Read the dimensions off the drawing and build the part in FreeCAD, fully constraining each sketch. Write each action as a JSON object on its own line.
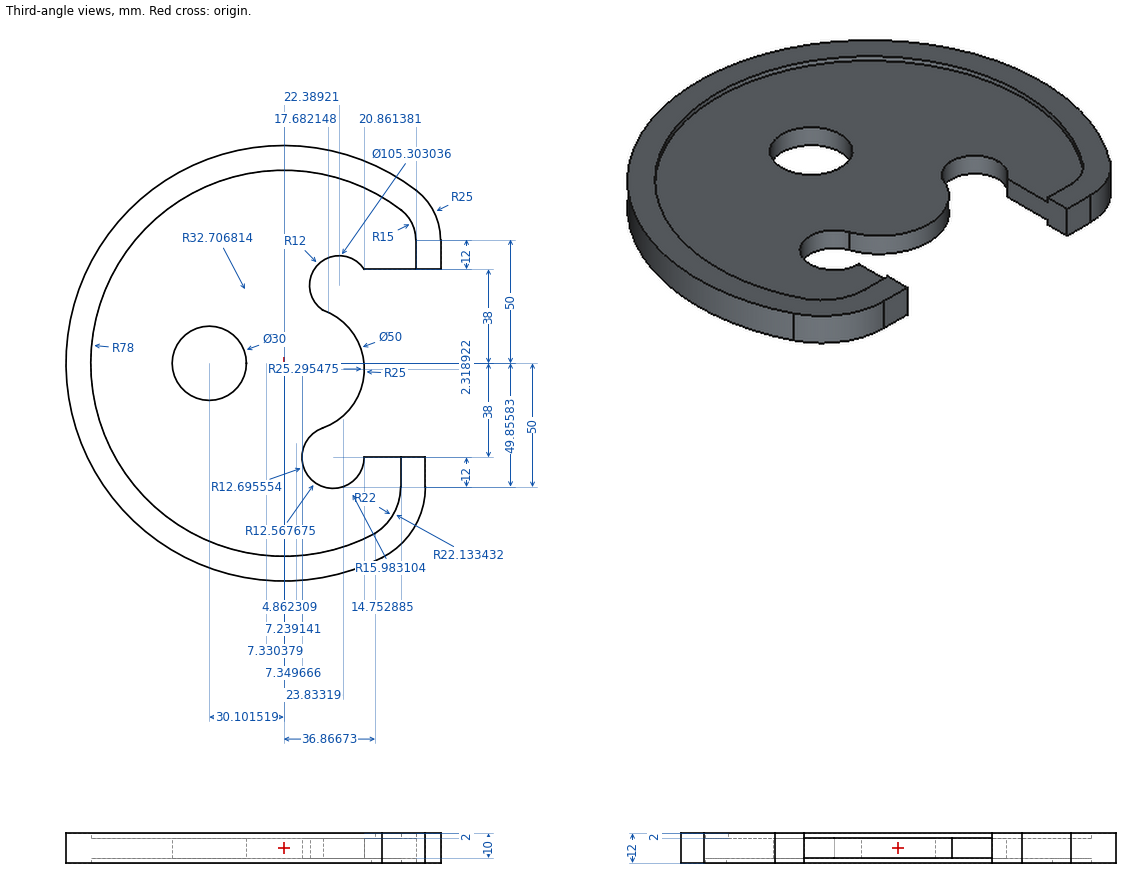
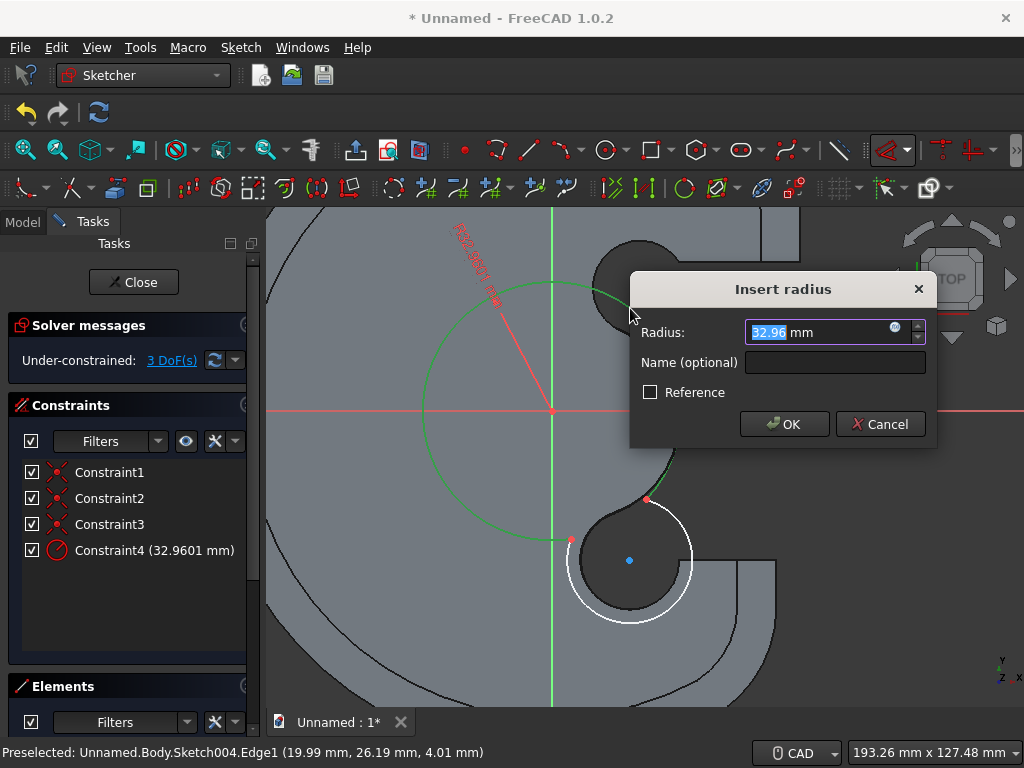
{"action": "type", "text": "32.706814"}
{"action": "key", "text": "Return"}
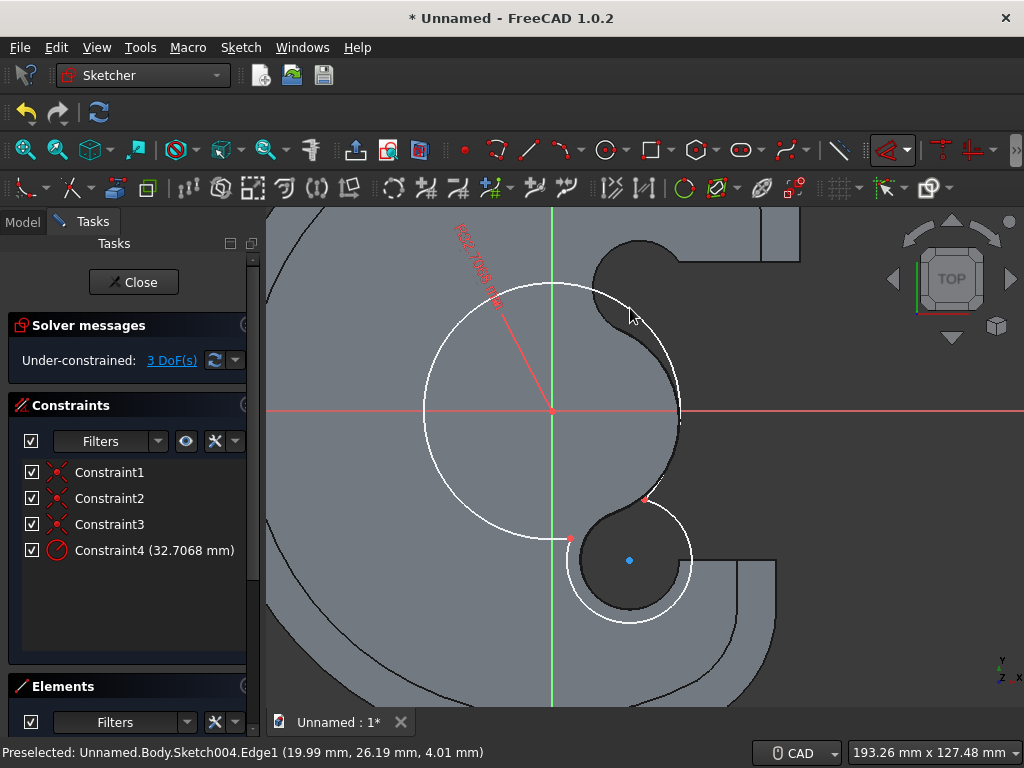
{"action": "left_click", "coordinate": [600, 616]}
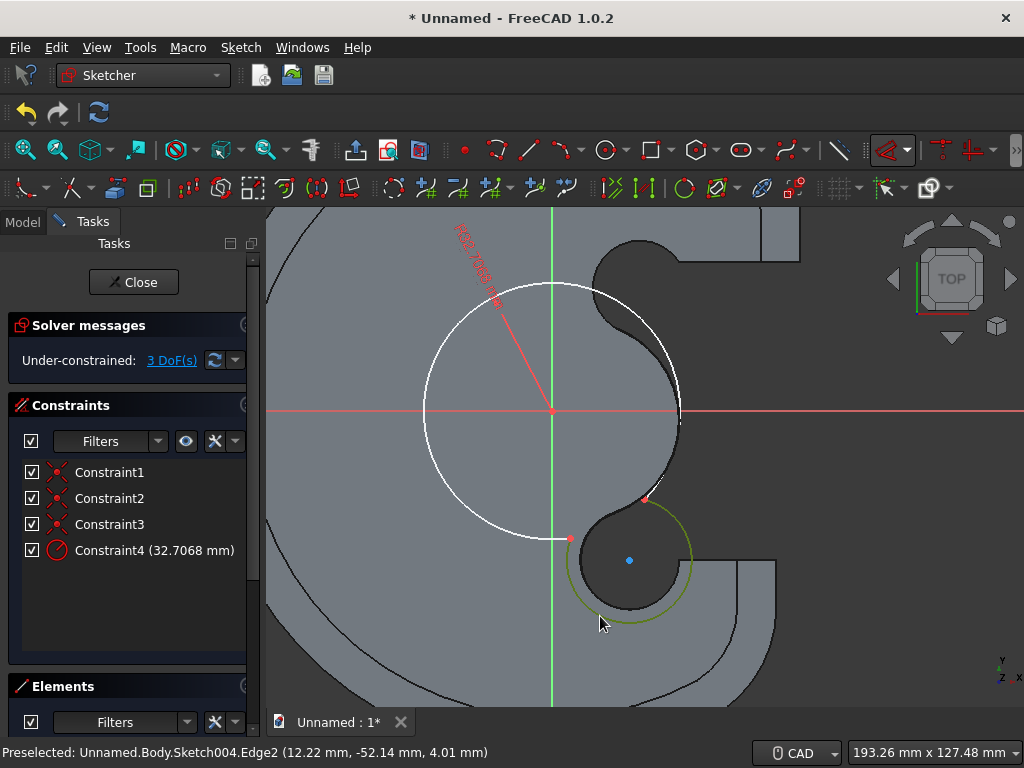
{"action": "left_click", "coordinate": [910, 150]}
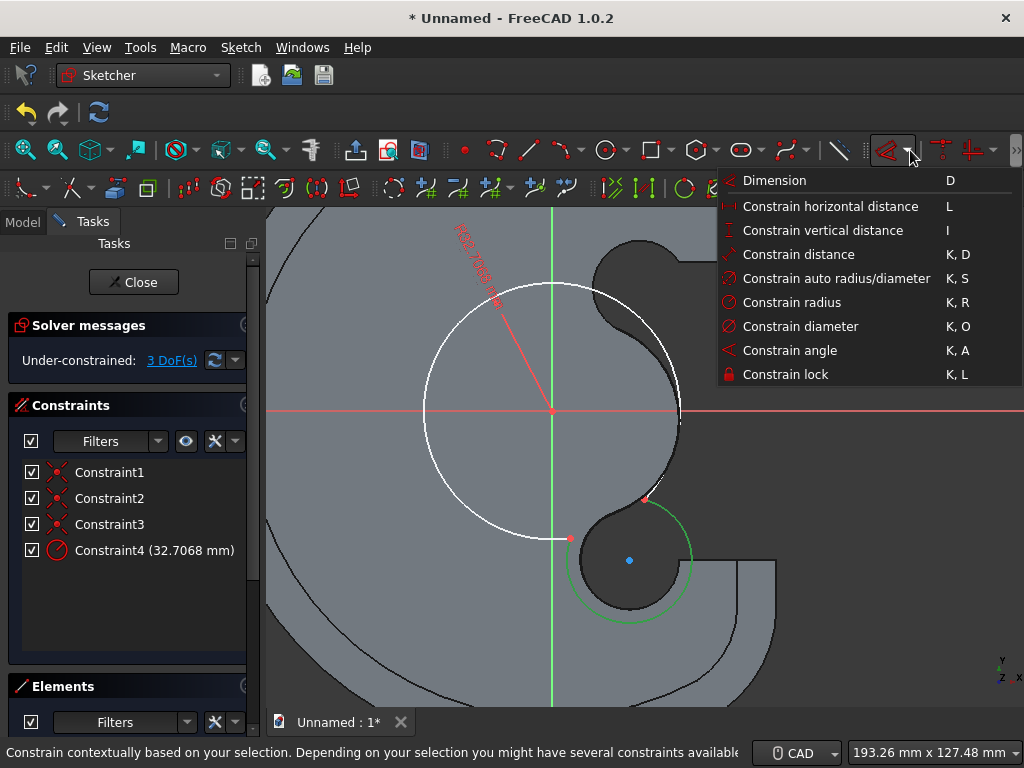
{"action": "left_click", "coordinate": [870, 302]}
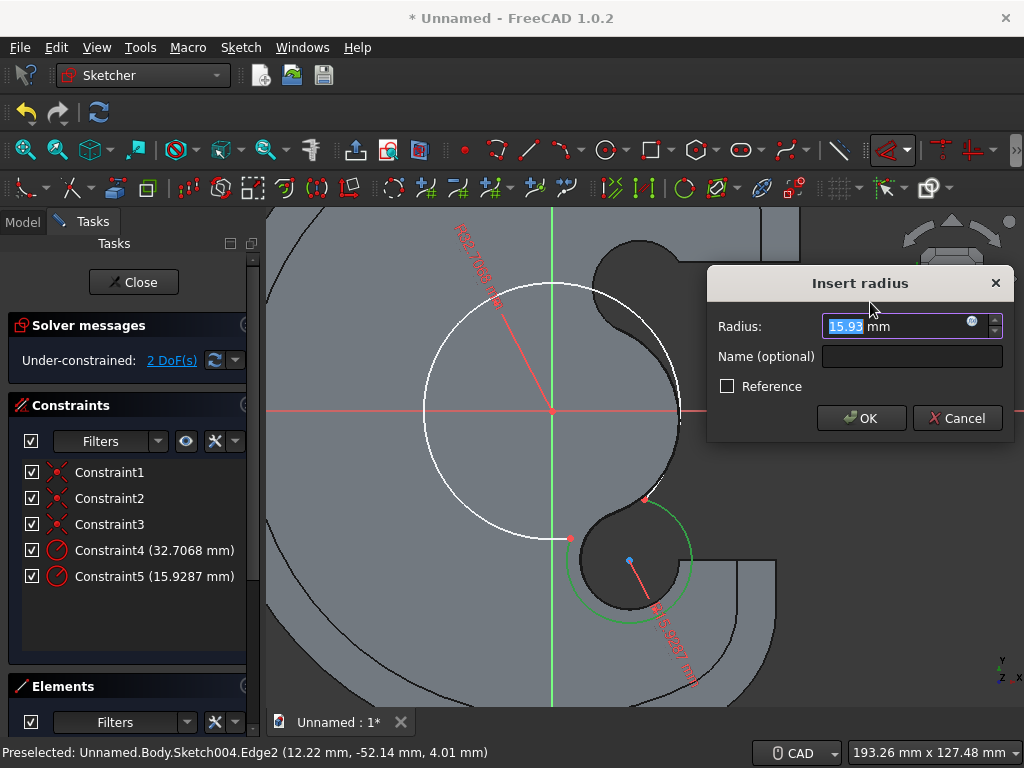
{"action": "type", "text": "15.983104"}
{"action": "key", "text": "Return"}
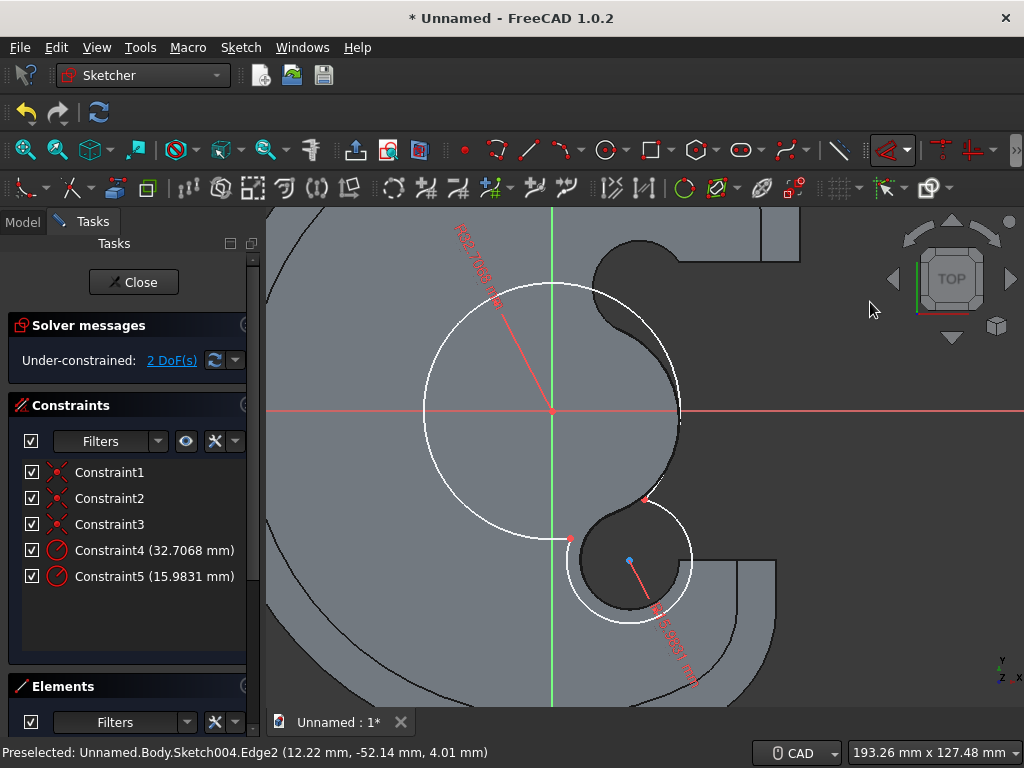
{"action": "left_click", "coordinate": [645, 500]}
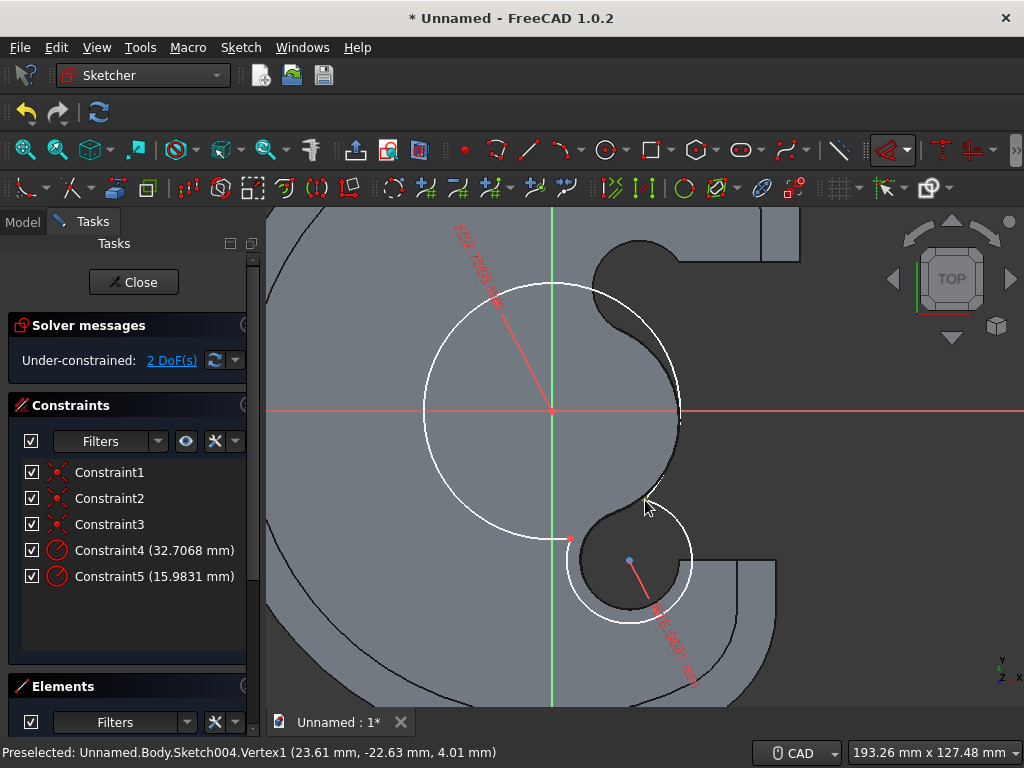
{"action": "key", "text": "l"}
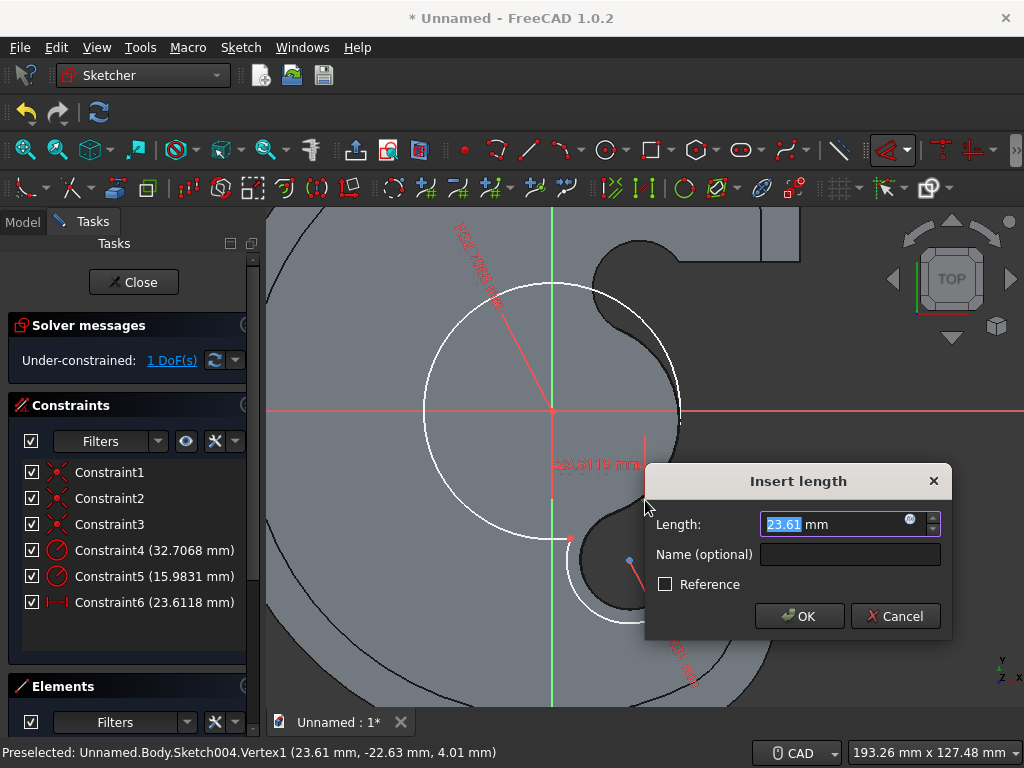
{"action": "type", "text": "23.83319"}
{"action": "key", "text": "Return"}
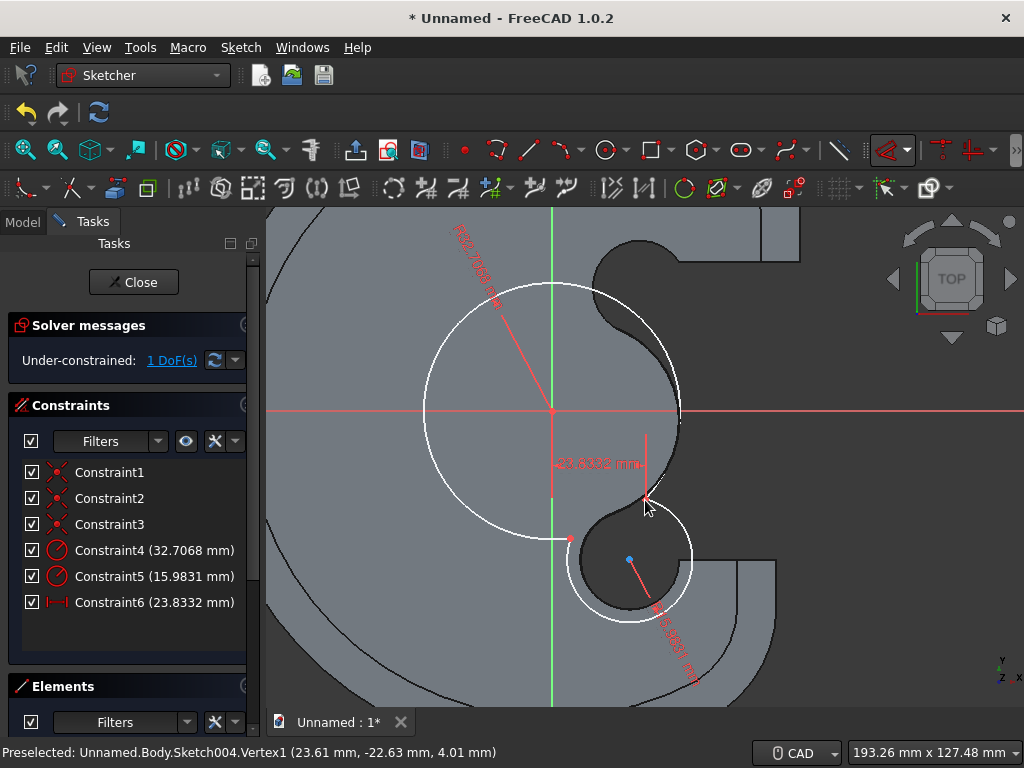
{"action": "scroll", "coordinate": [571, 538], "scroll_direction": "up", "scroll_amount": 4}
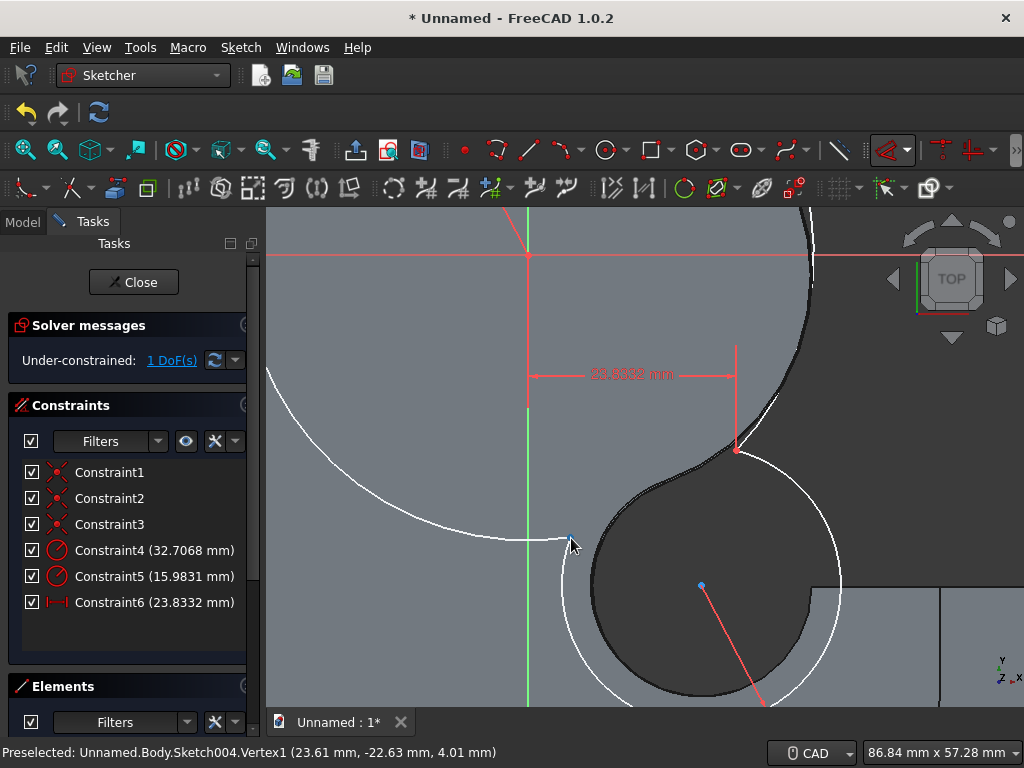
{"action": "left_click", "coordinate": [570, 537]}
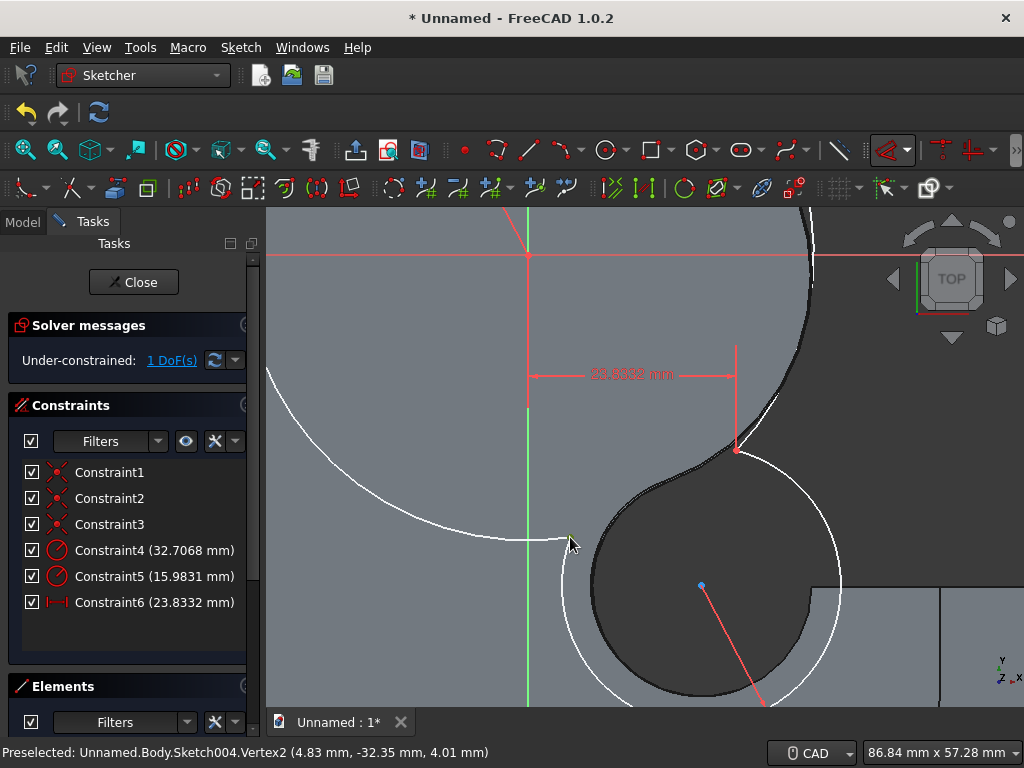
{"action": "key", "text": "l"}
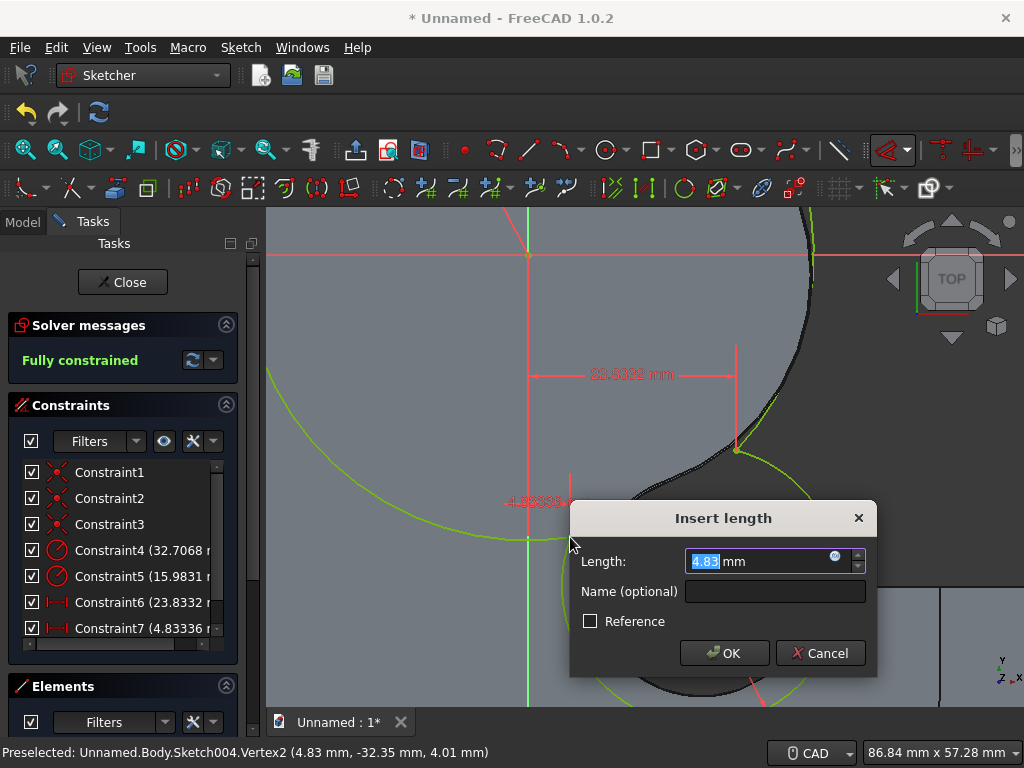
{"action": "type", "text": "4.862309"}
{"action": "key", "text": "Return"}